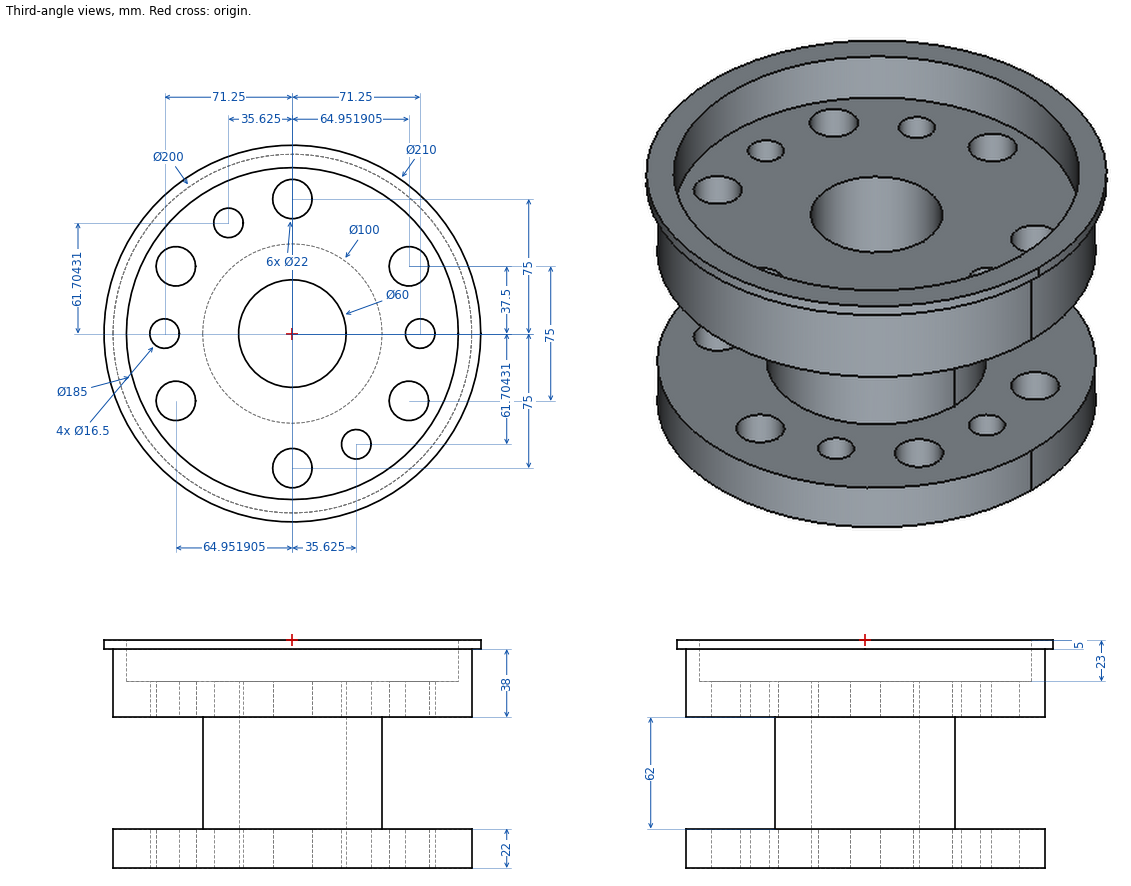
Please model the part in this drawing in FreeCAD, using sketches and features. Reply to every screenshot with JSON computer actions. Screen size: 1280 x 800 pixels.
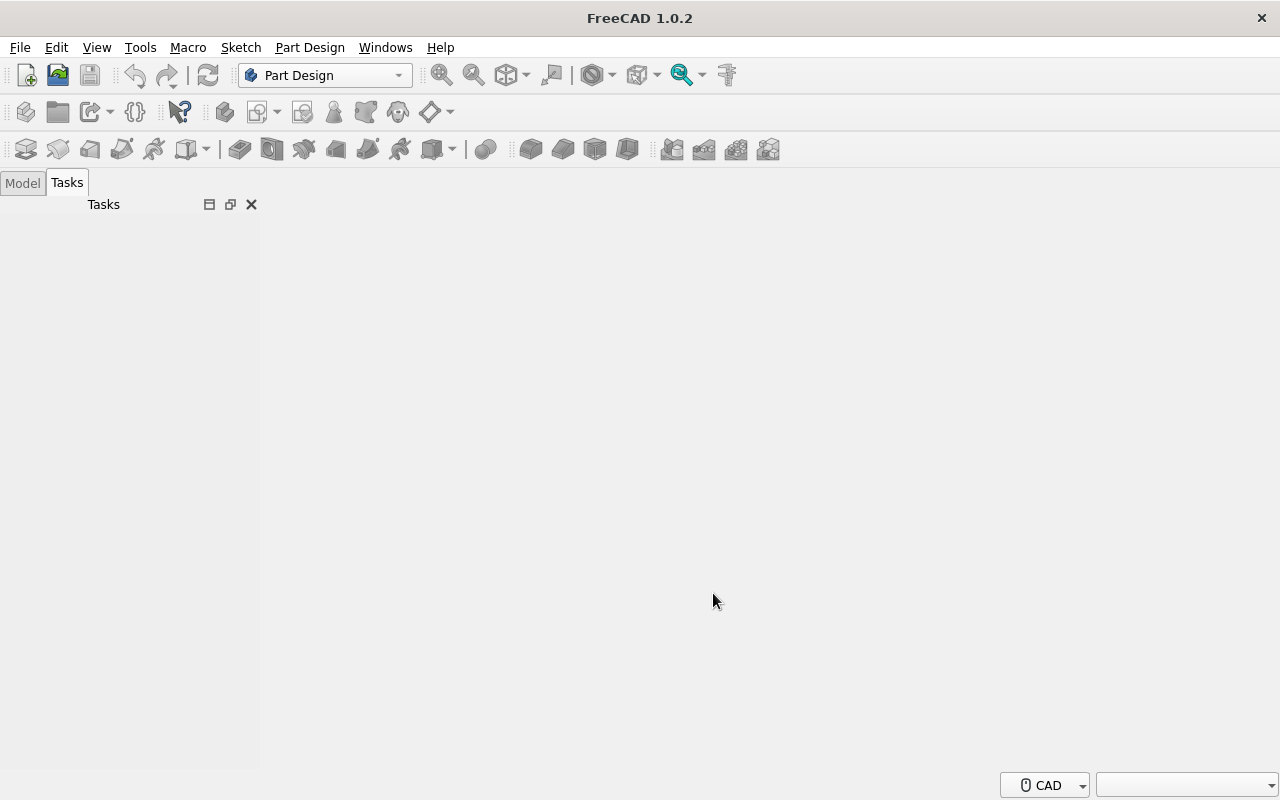
{"action": "left_click", "coordinate": [26, 76]}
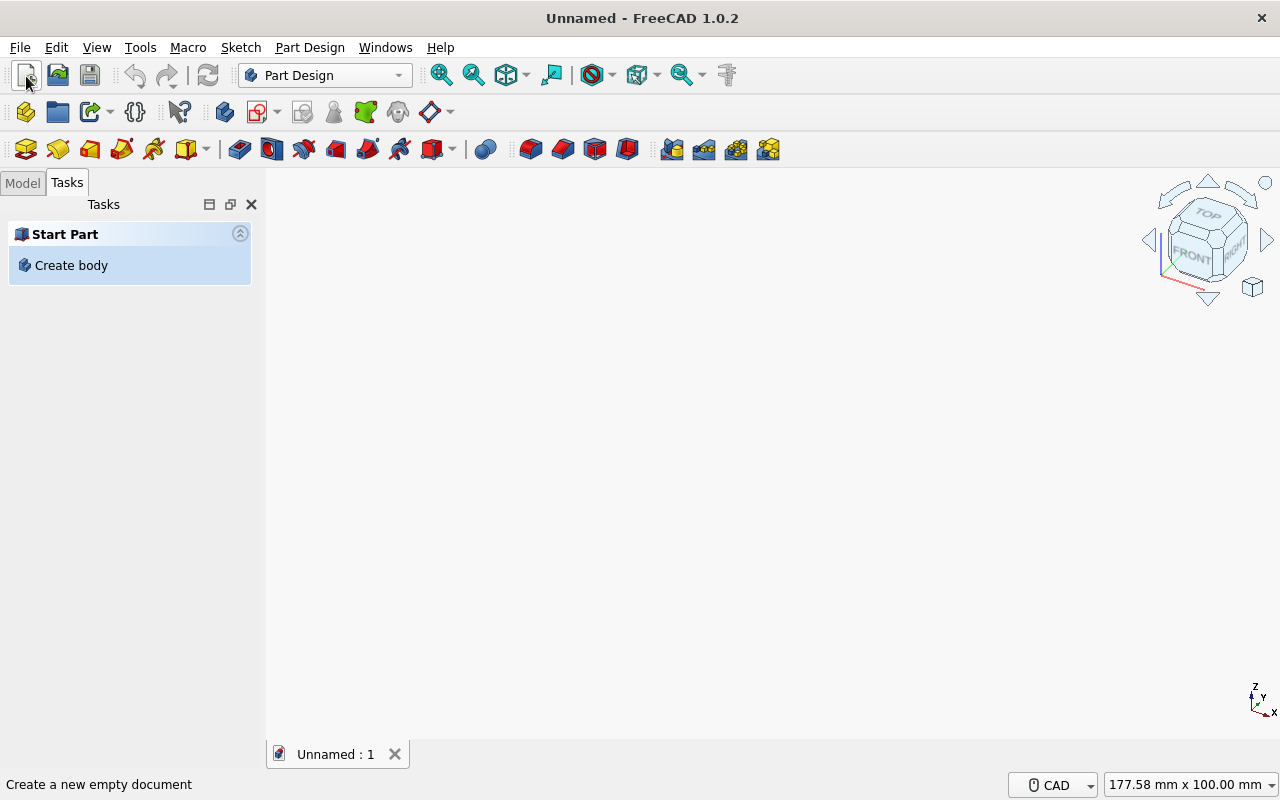
{"action": "left_click", "coordinate": [258, 112]}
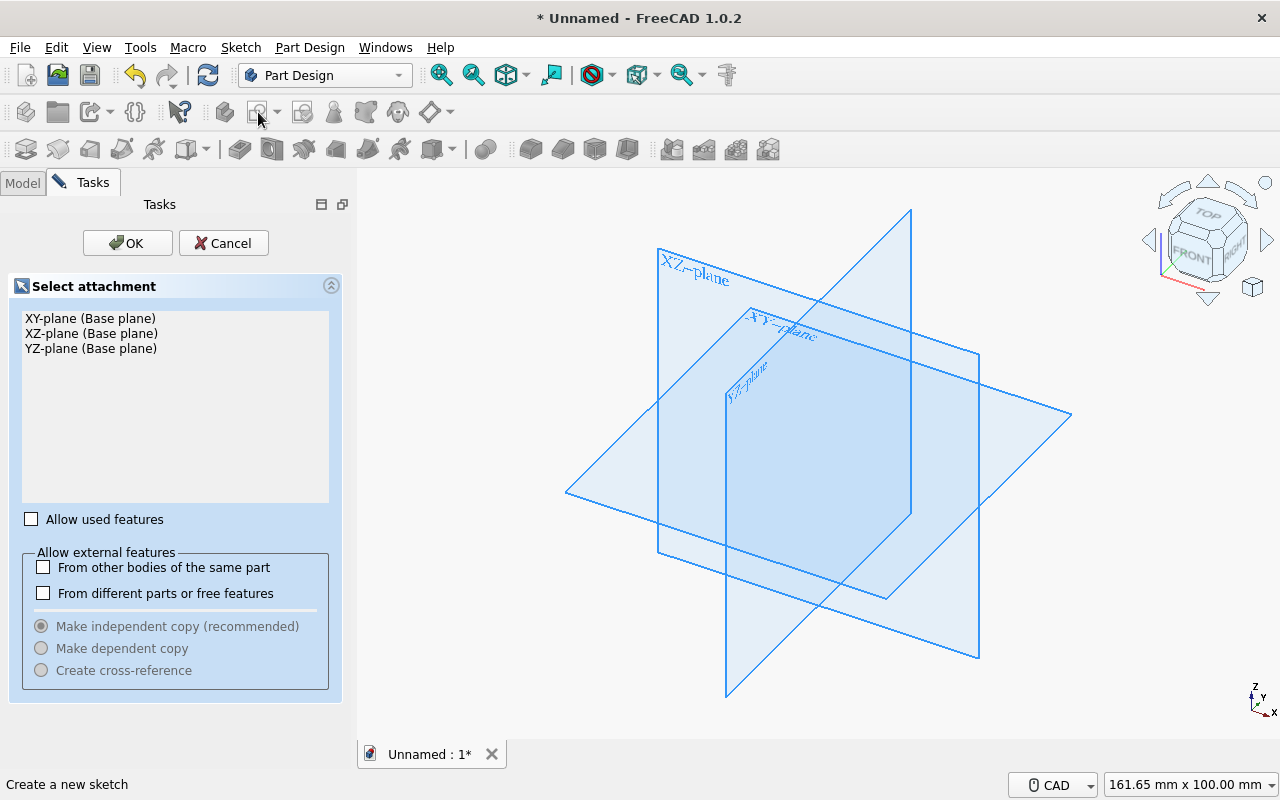
{"action": "left_click", "coordinate": [82, 318]}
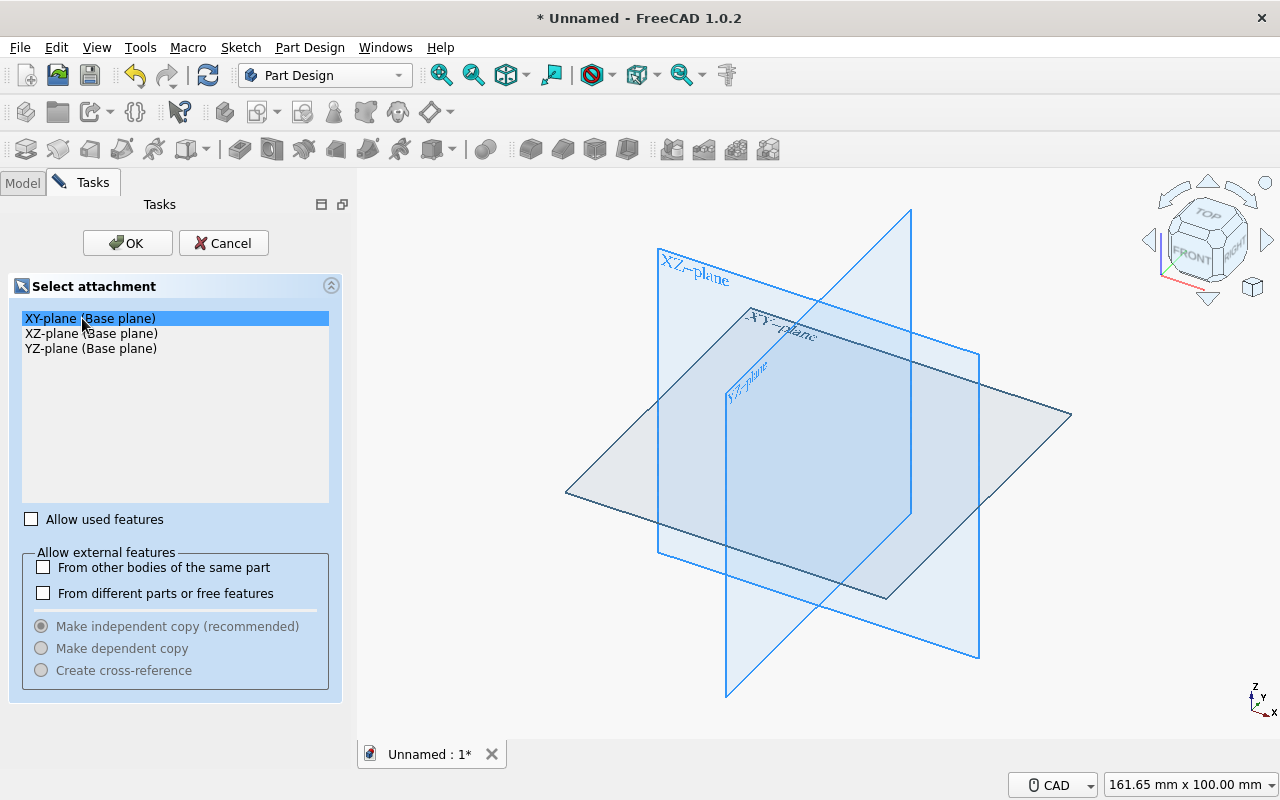
{"action": "left_click", "coordinate": [128, 243]}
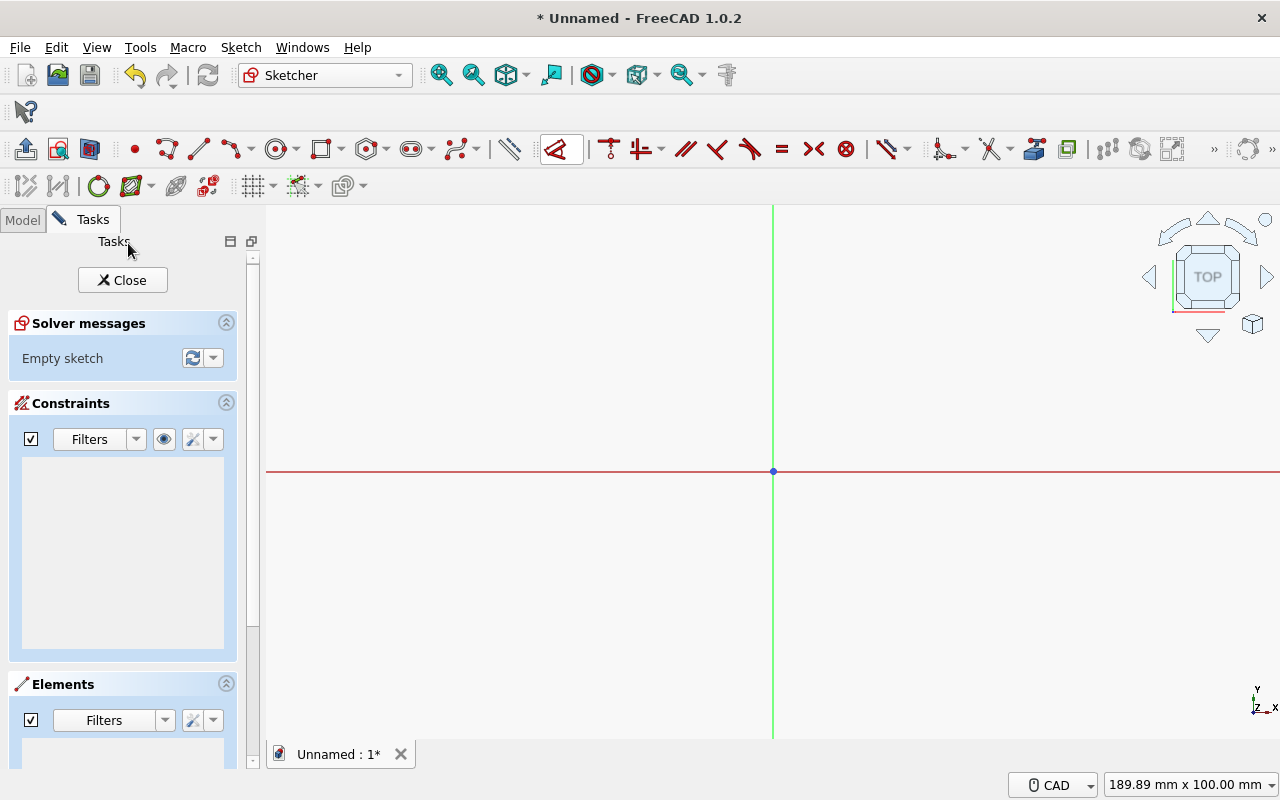
{"action": "scroll", "coordinate": [675, 472], "scroll_direction": "down", "scroll_amount": 6}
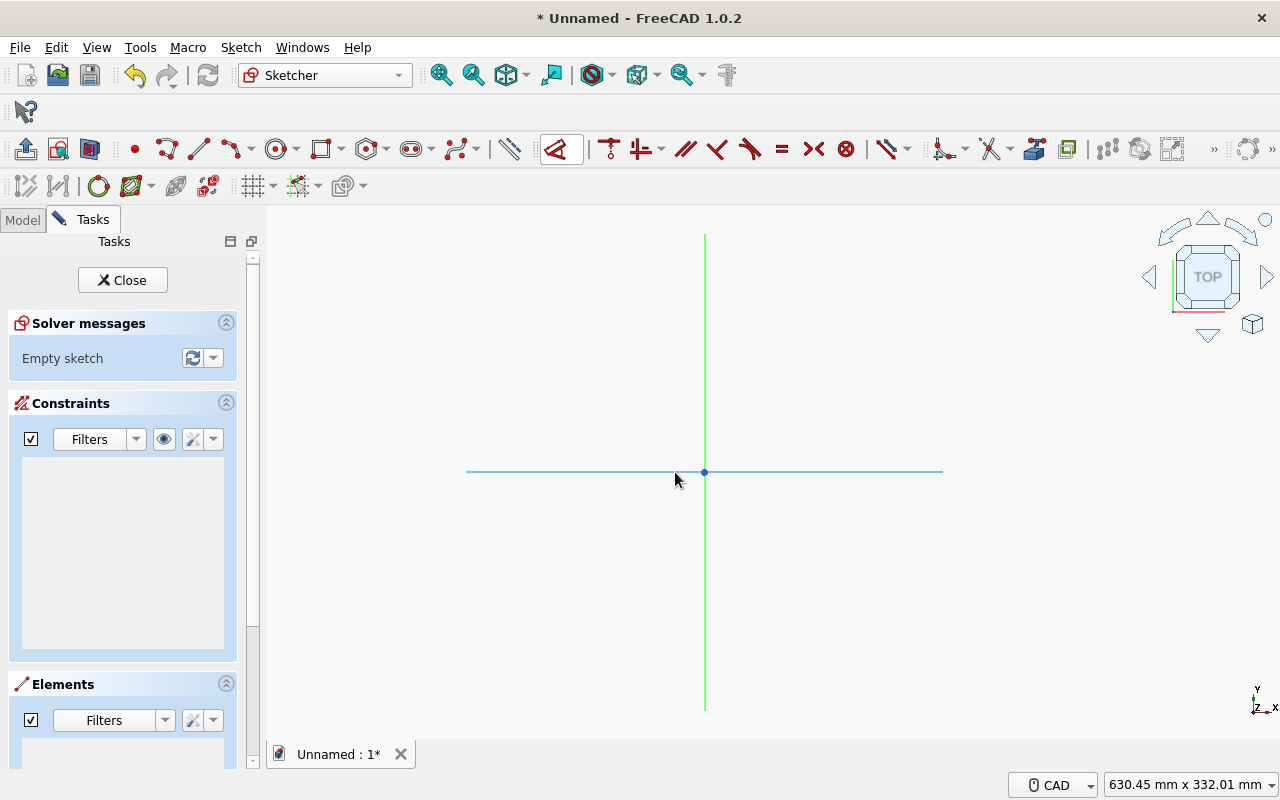
{"action": "left_click", "coordinate": [276, 150]}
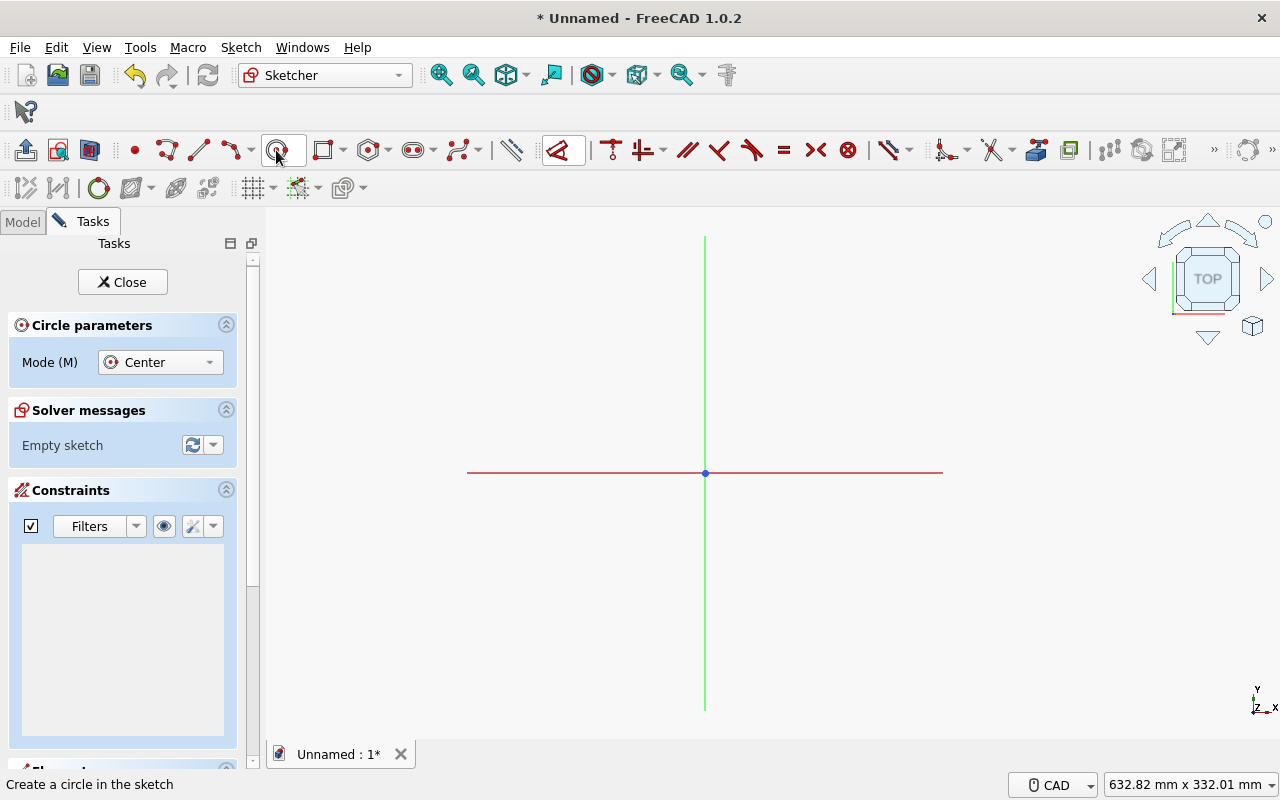
{"action": "left_click", "coordinate": [705, 473]}
{"action": "mouse_move", "coordinate": [824, 354]}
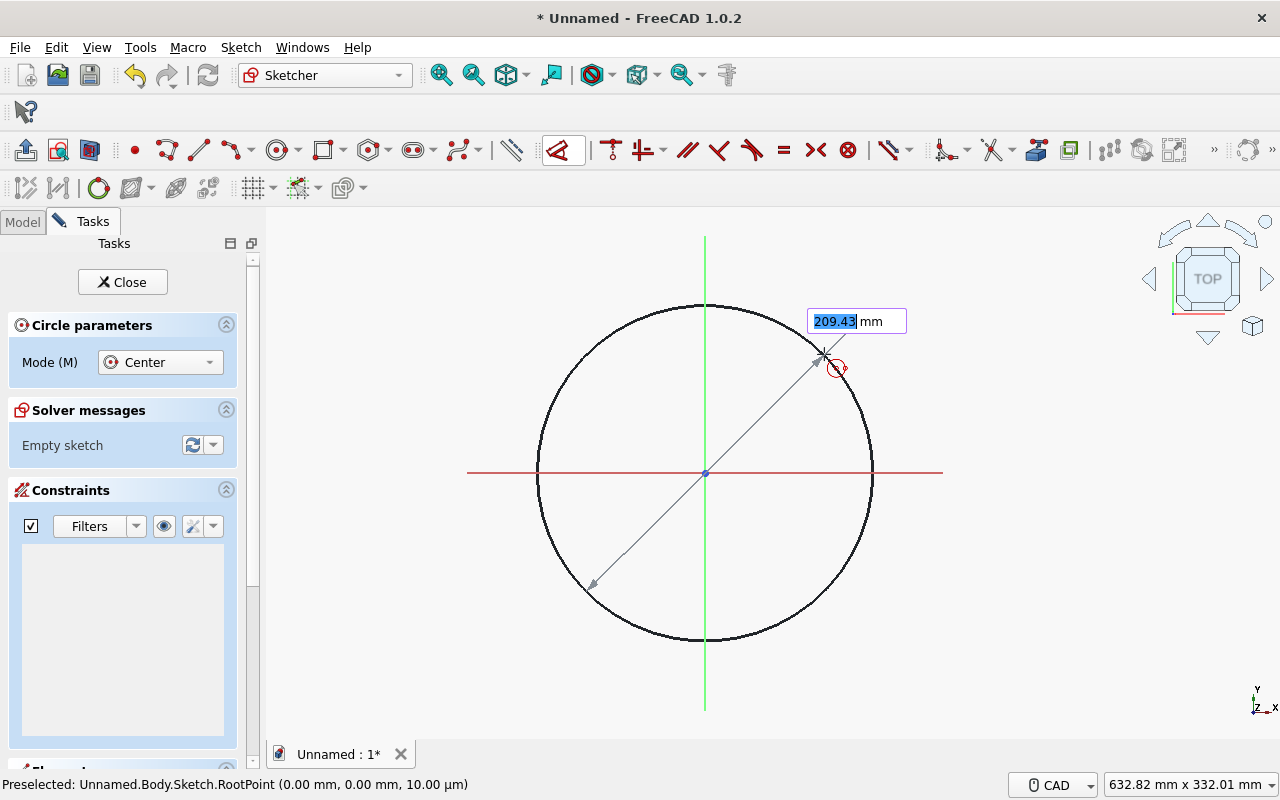
{"action": "type", "text": "210"}
{"action": "key", "text": "Return"}
{"action": "key", "text": "Escape"}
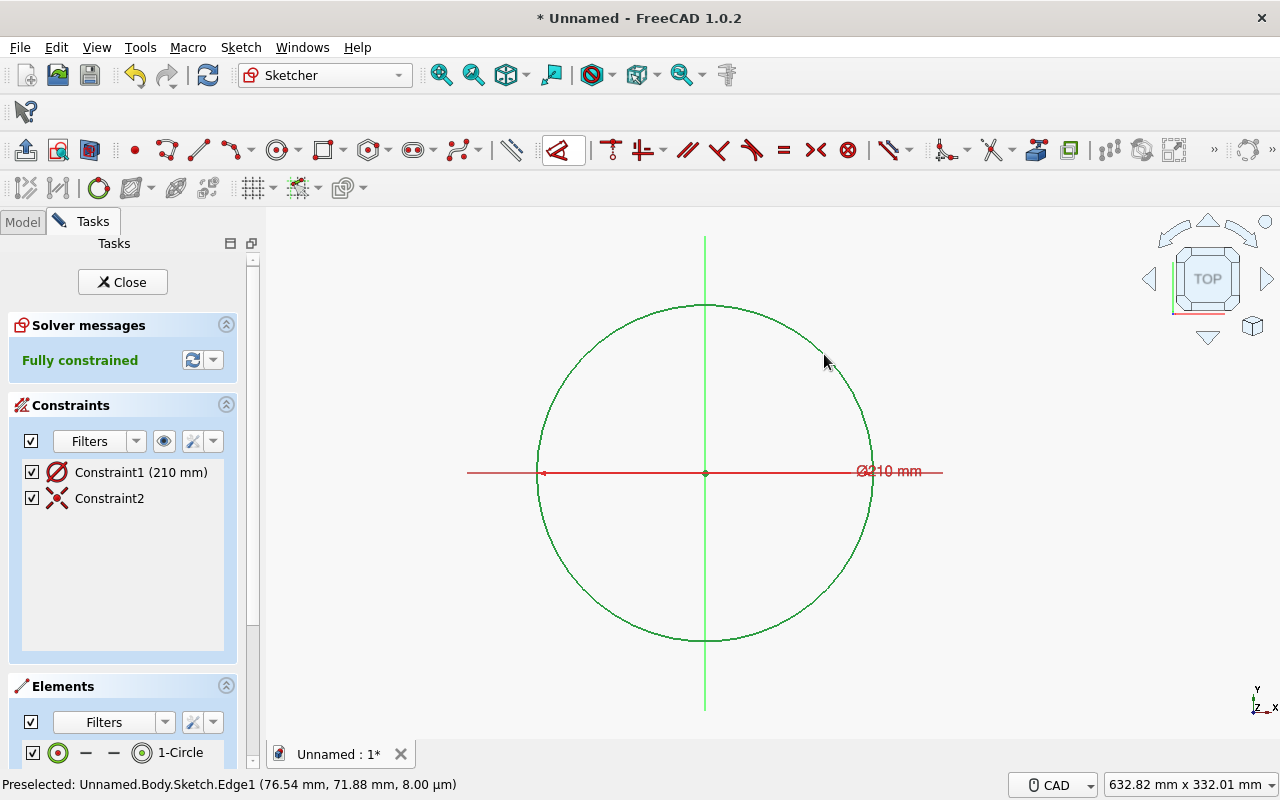
{"action": "left_click", "coordinate": [123, 282]}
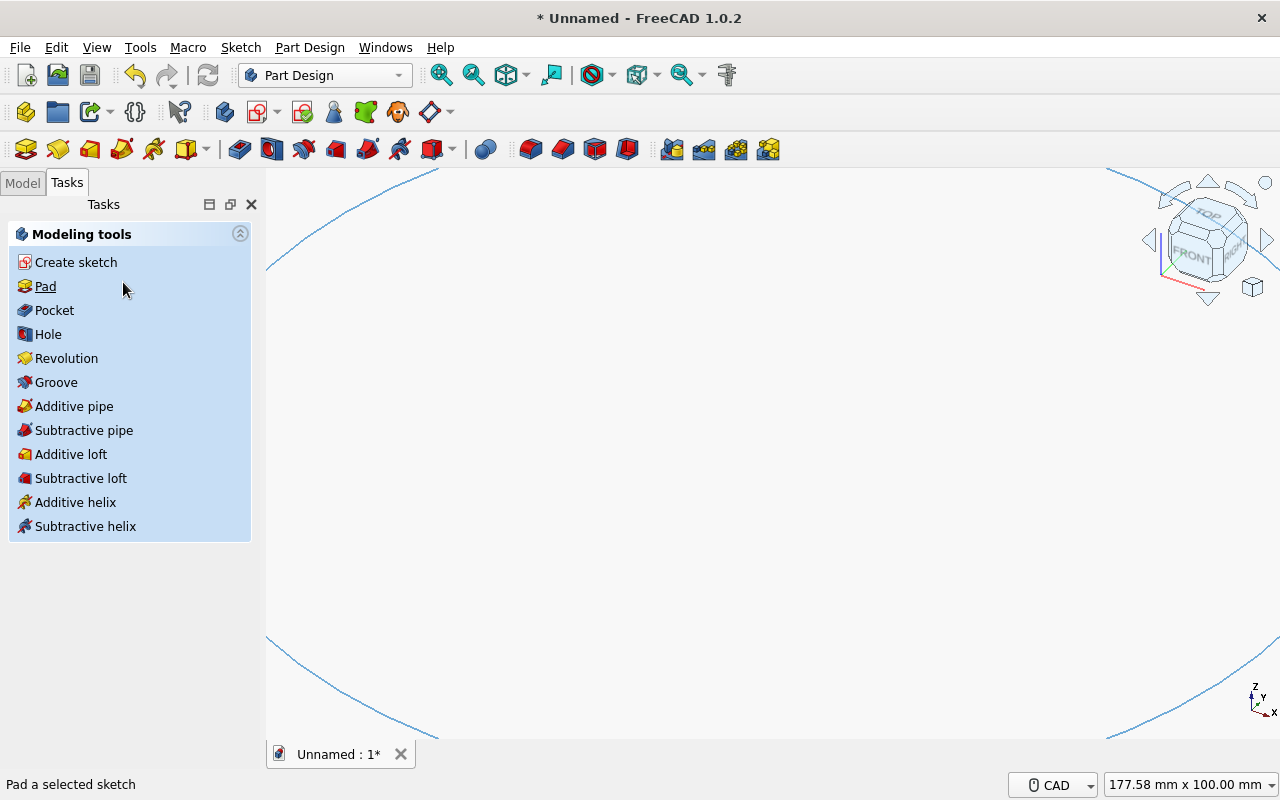
{"action": "left_click", "coordinate": [26, 150]}